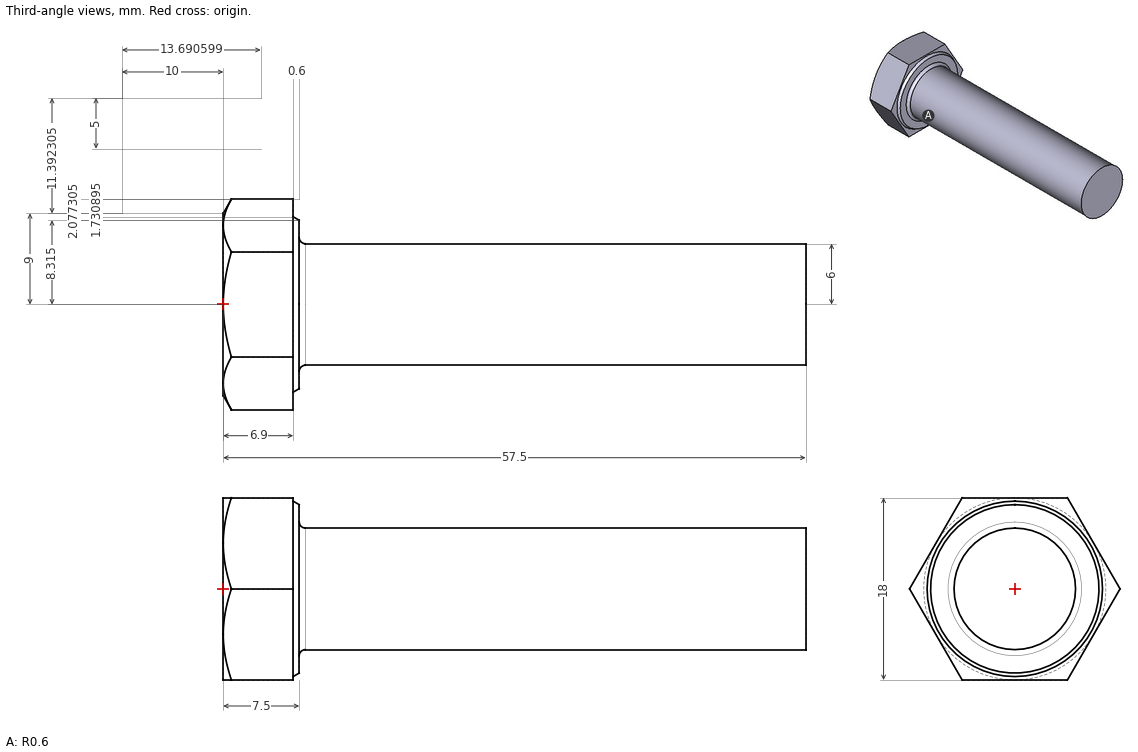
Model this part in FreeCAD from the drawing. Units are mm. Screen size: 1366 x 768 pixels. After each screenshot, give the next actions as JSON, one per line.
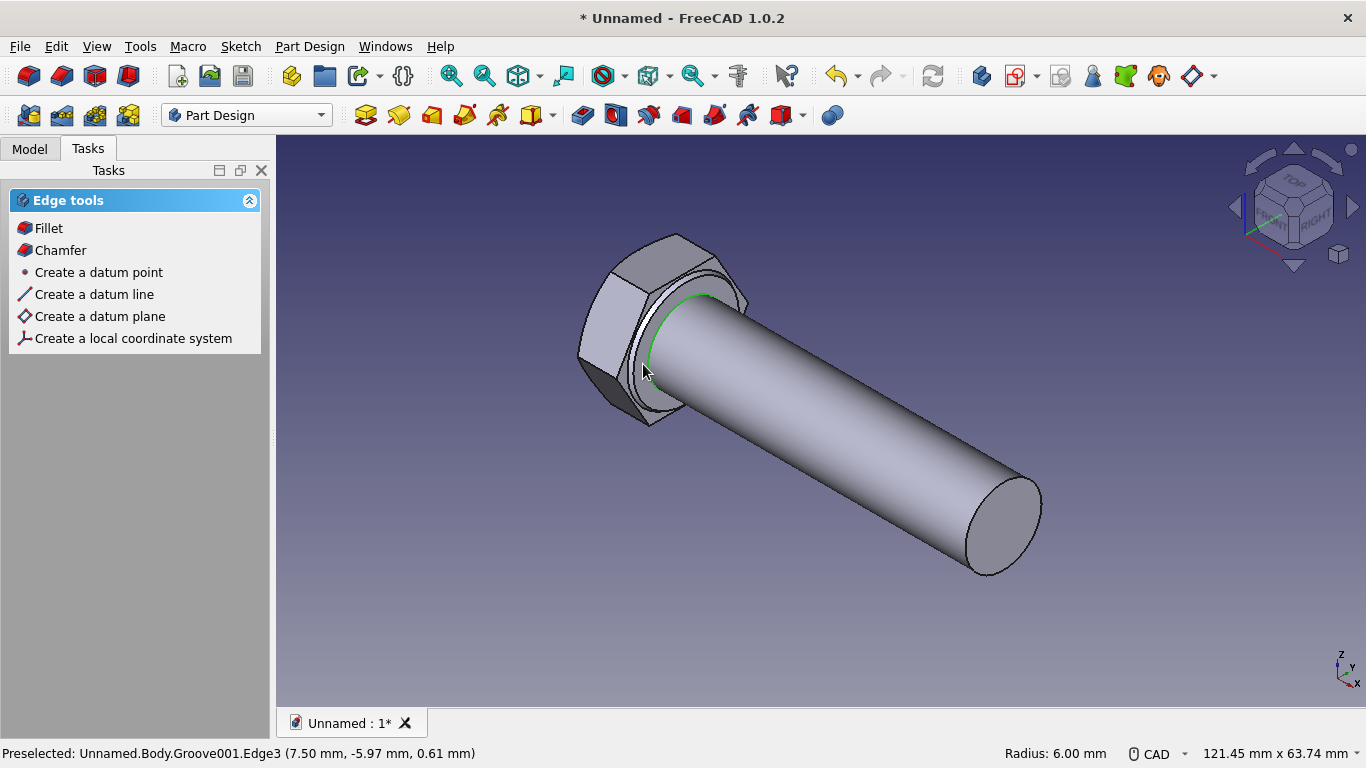
{"action": "left_click", "coordinate": [29, 76]}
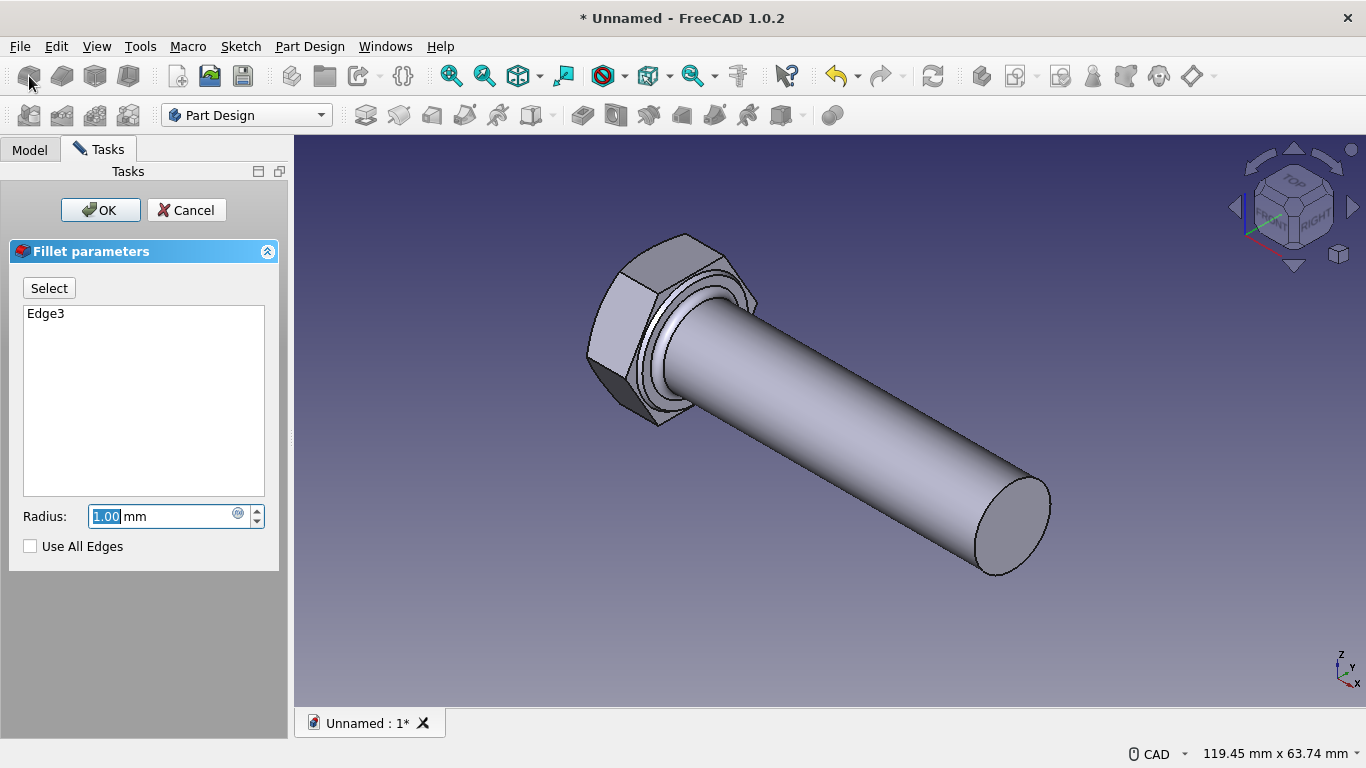
{"action": "type", "text": "0.6"}
{"action": "key", "text": "Tab"}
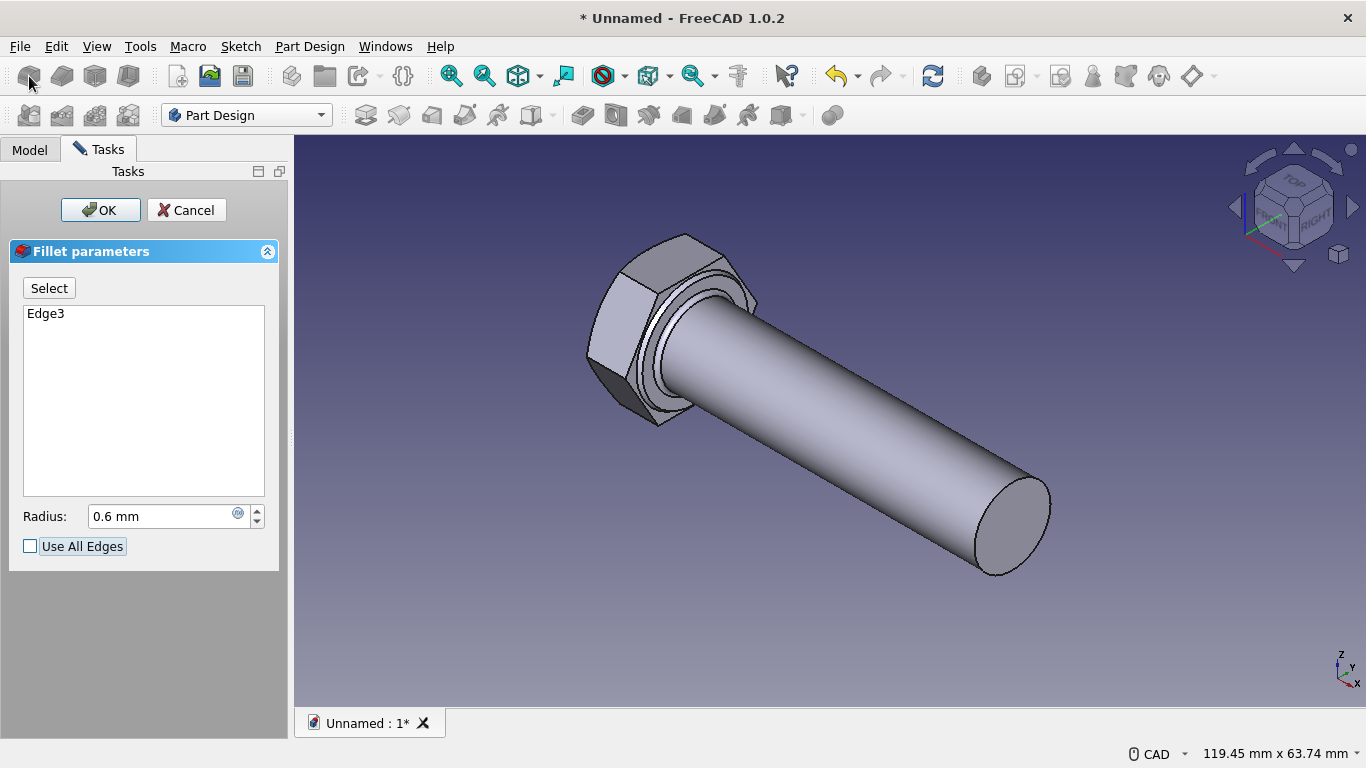
{"action": "left_click", "coordinate": [101, 210]}